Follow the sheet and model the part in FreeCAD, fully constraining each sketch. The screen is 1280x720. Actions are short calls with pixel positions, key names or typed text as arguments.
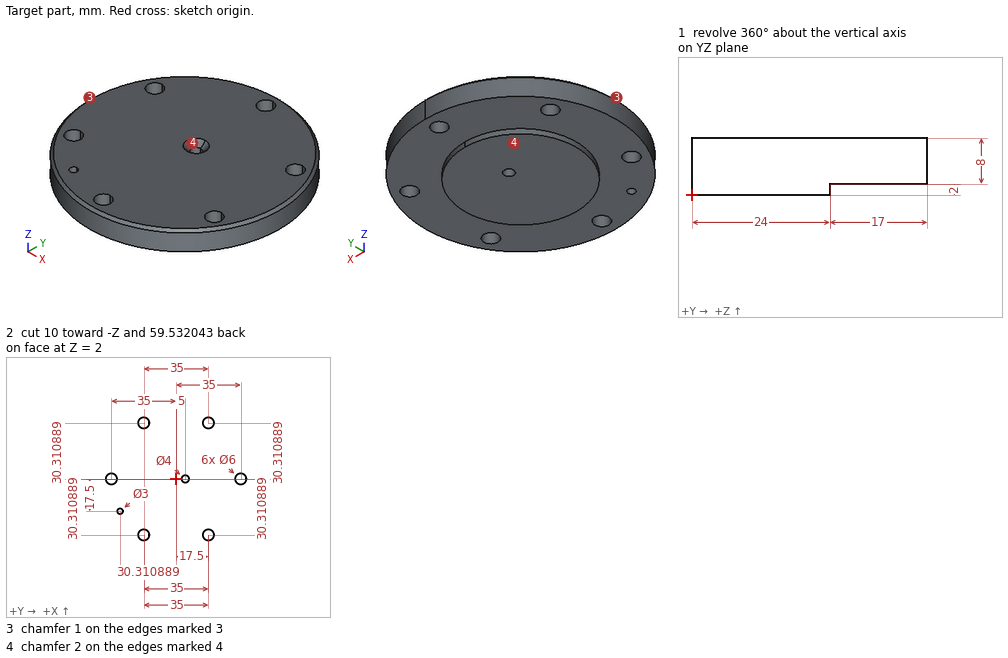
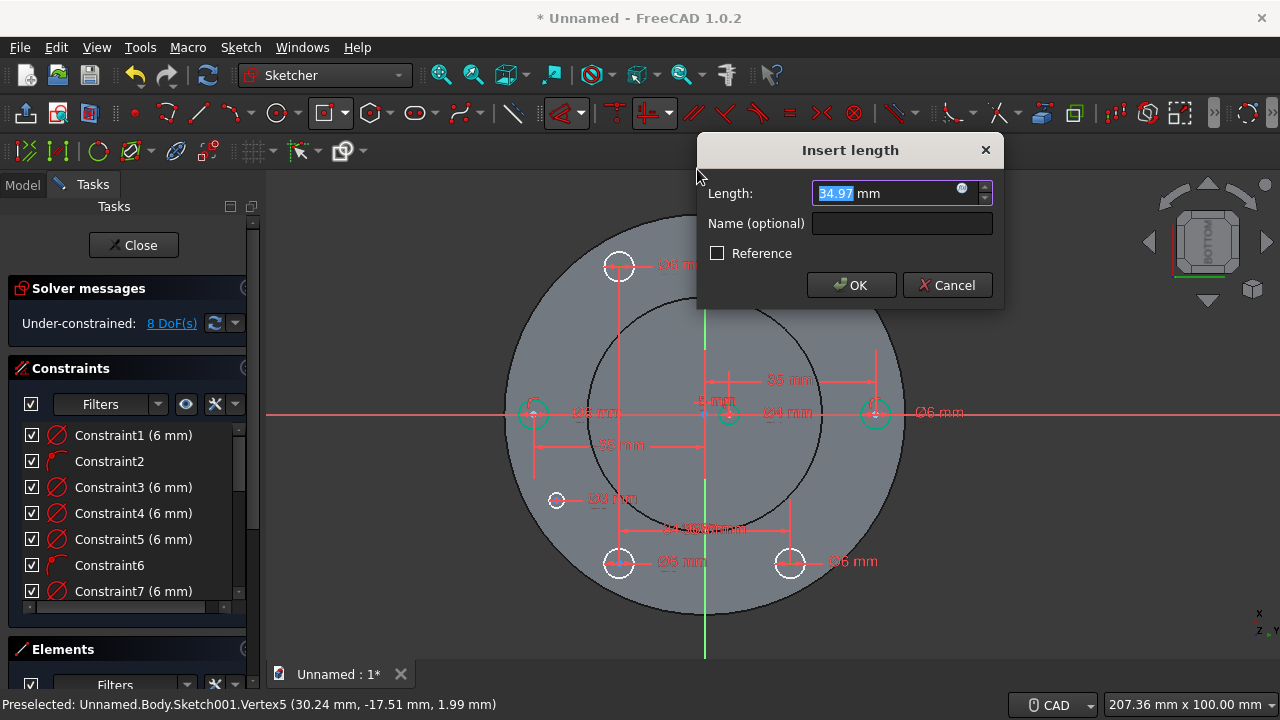
text(35)
key(Return)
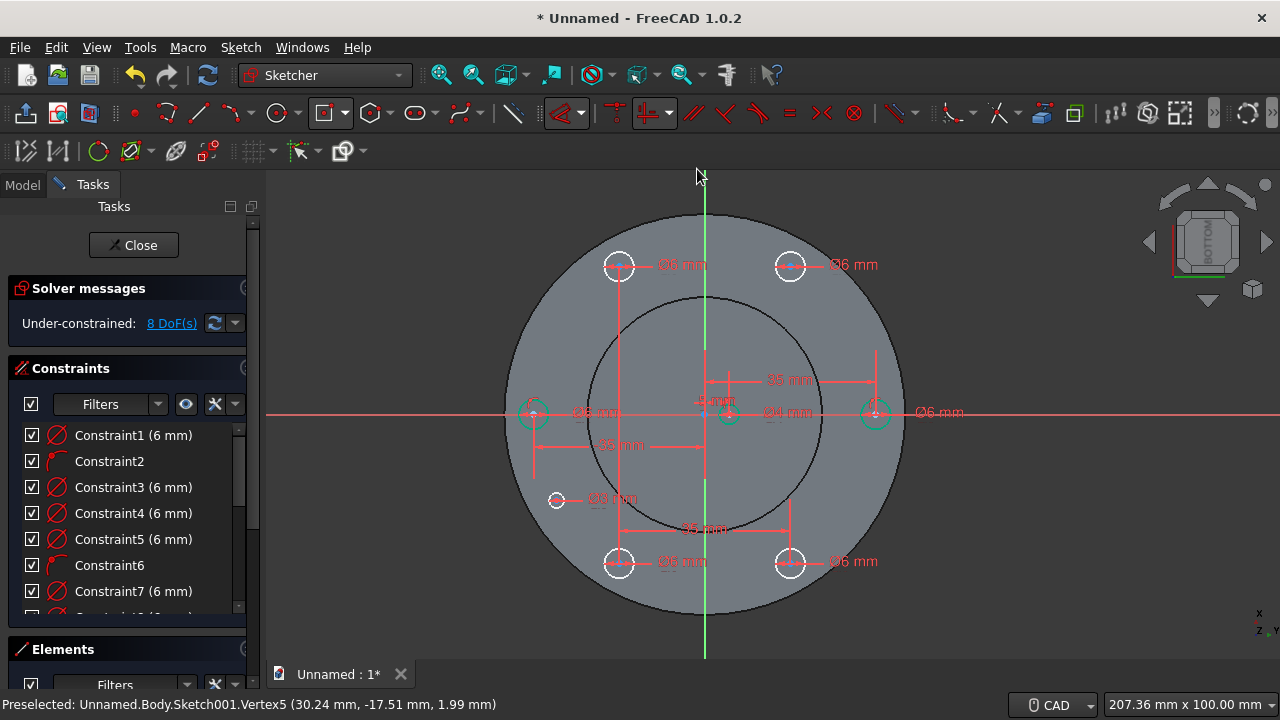
click(619, 267)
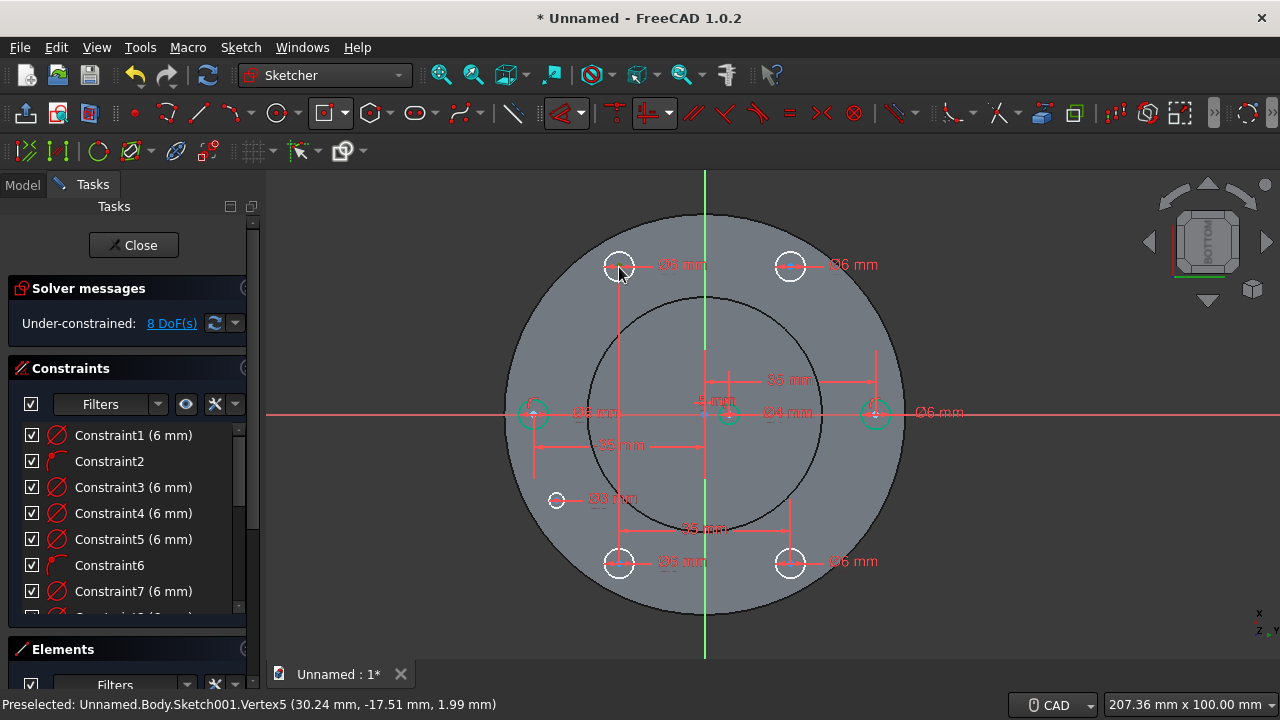
click(790, 267)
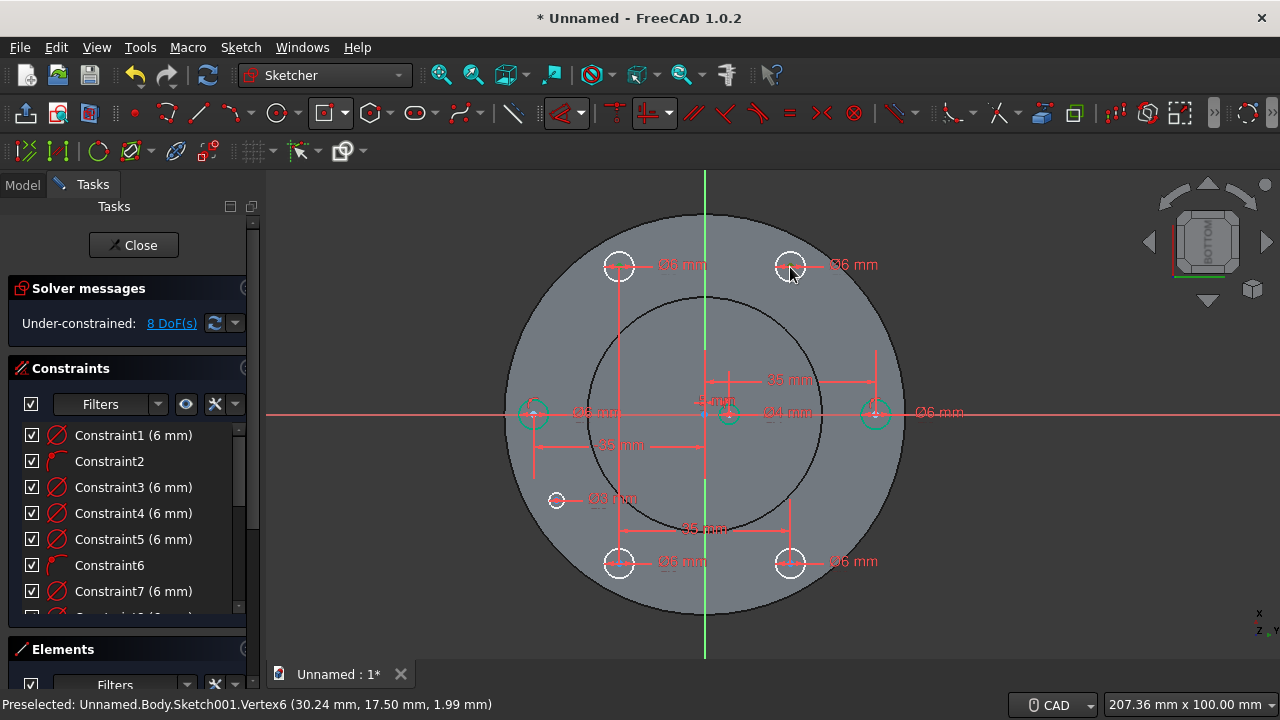
key(l)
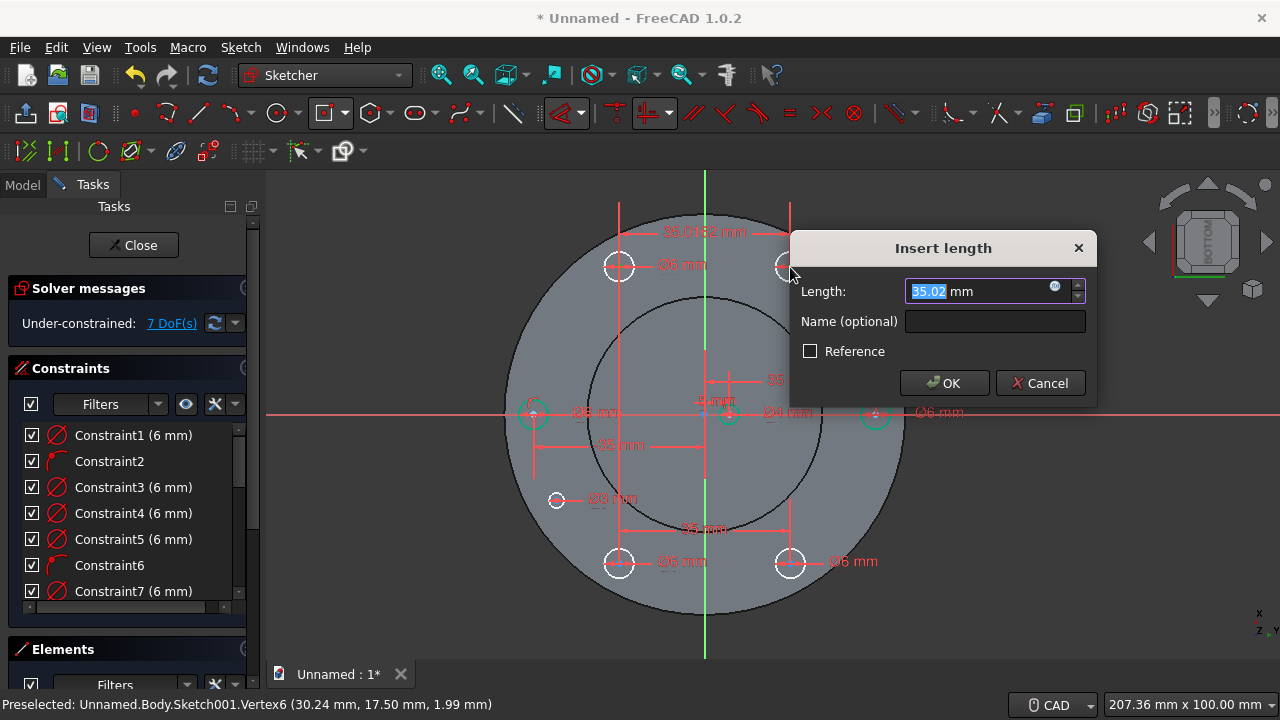
text(35)
key(Return)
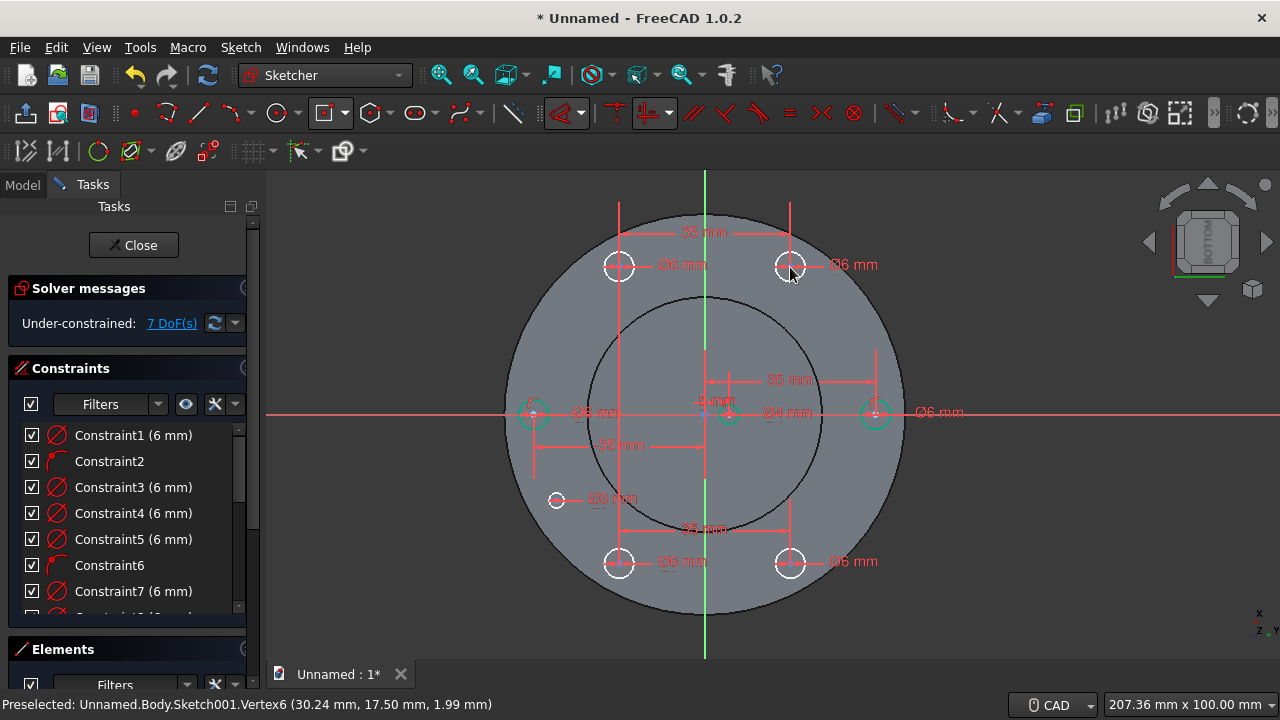
click(790, 564)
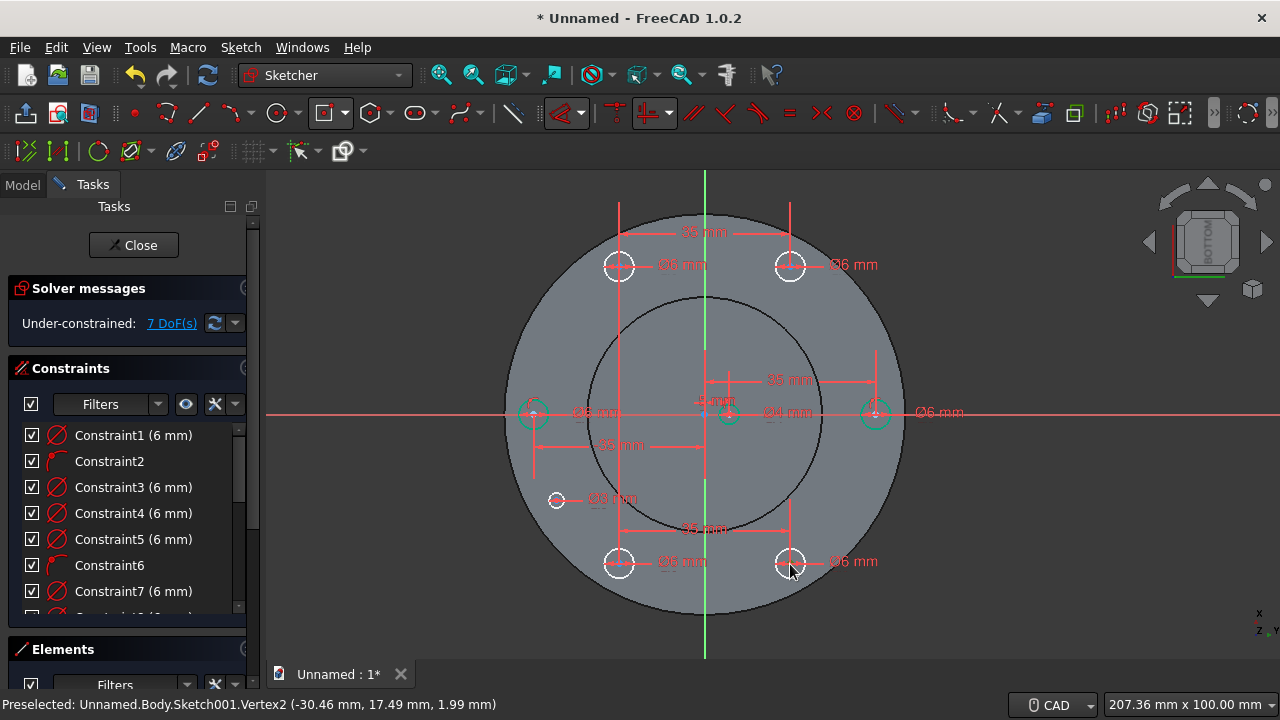
key(l)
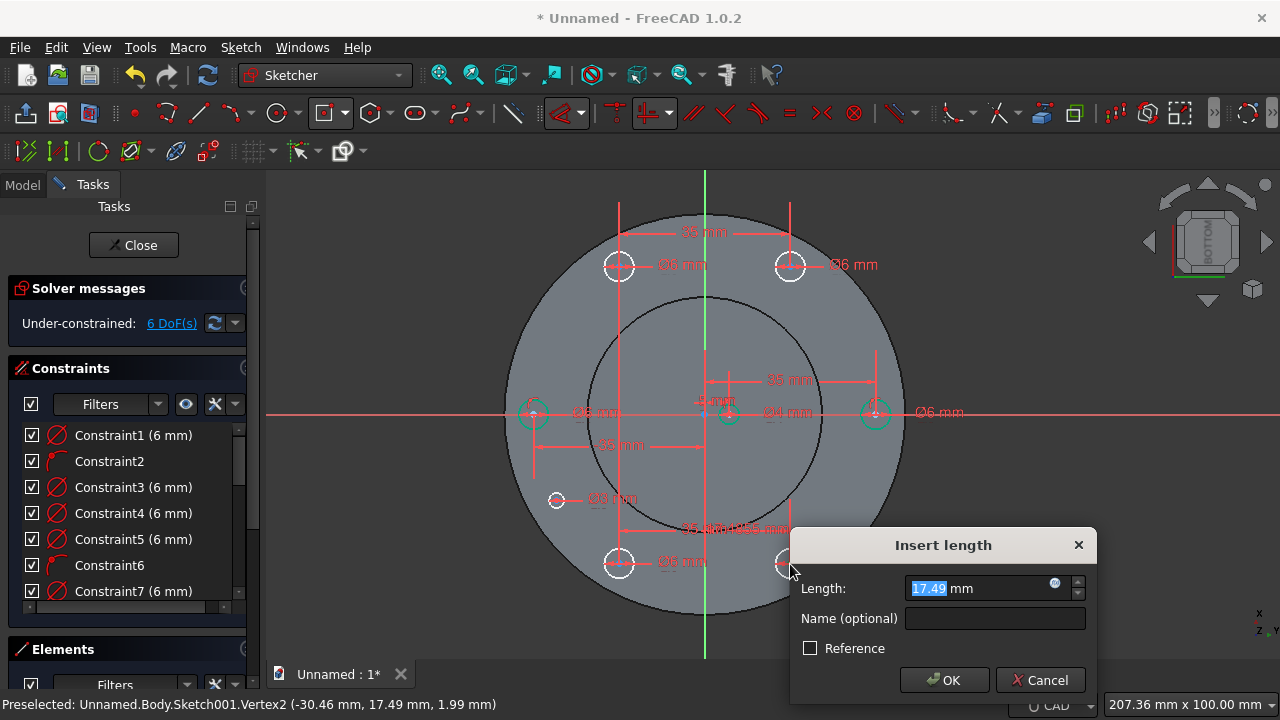
text(17.5)
key(Return)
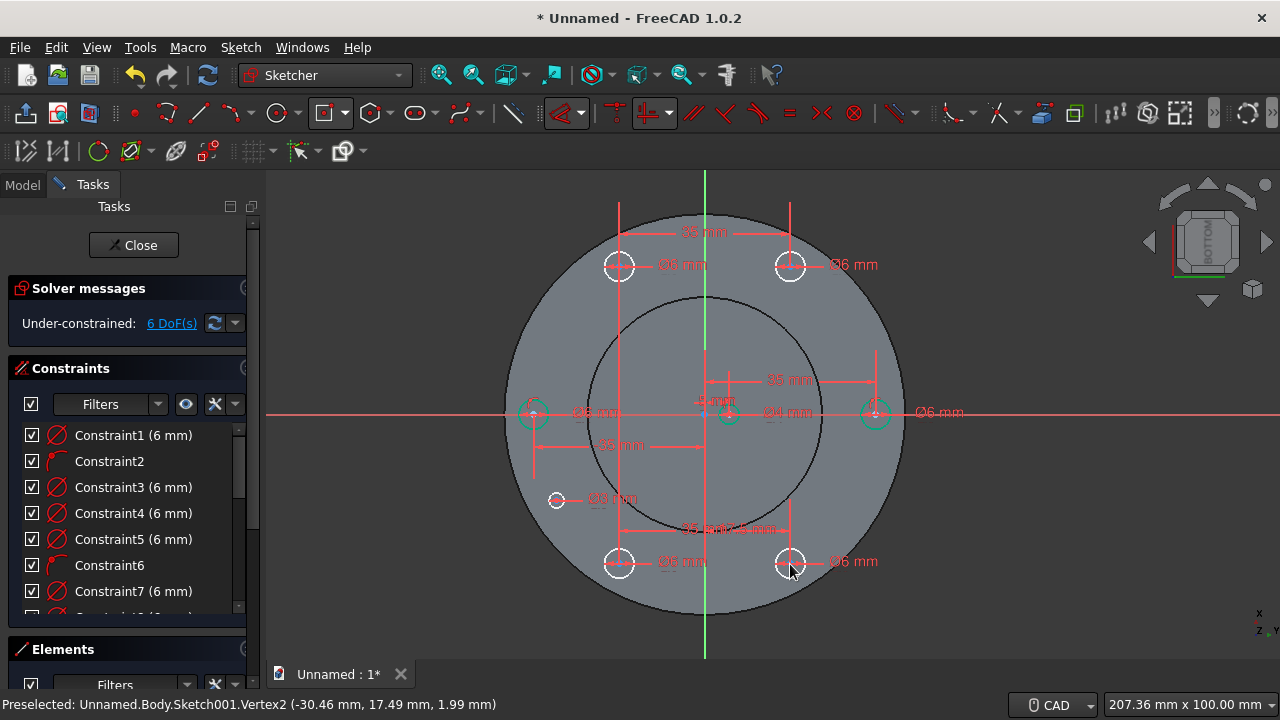
click(557, 501)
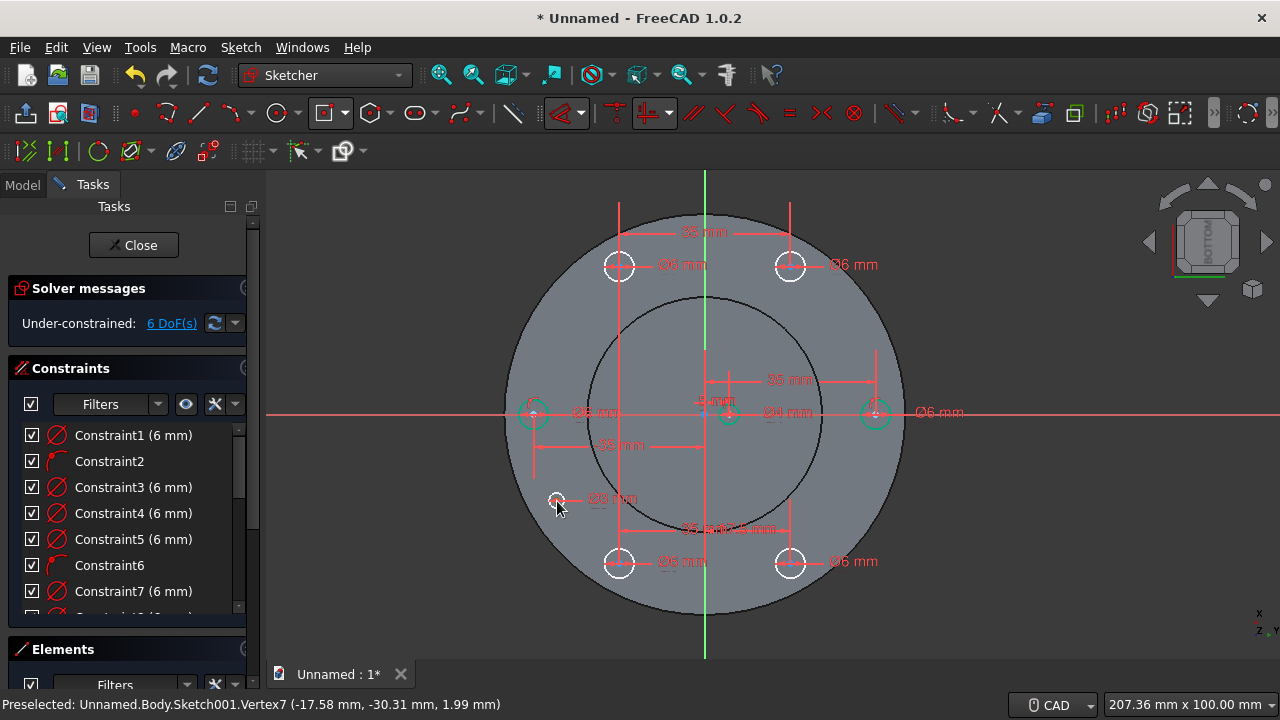
key(i)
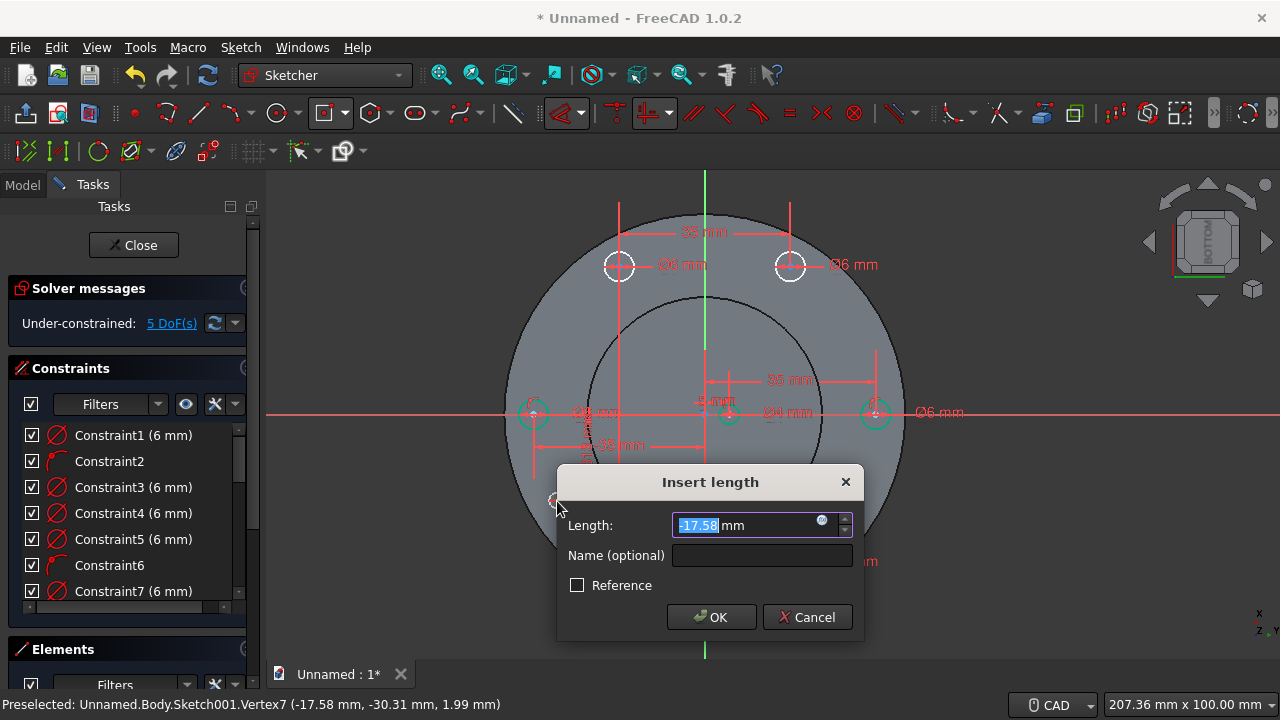
text(-17.5)
key(Return)